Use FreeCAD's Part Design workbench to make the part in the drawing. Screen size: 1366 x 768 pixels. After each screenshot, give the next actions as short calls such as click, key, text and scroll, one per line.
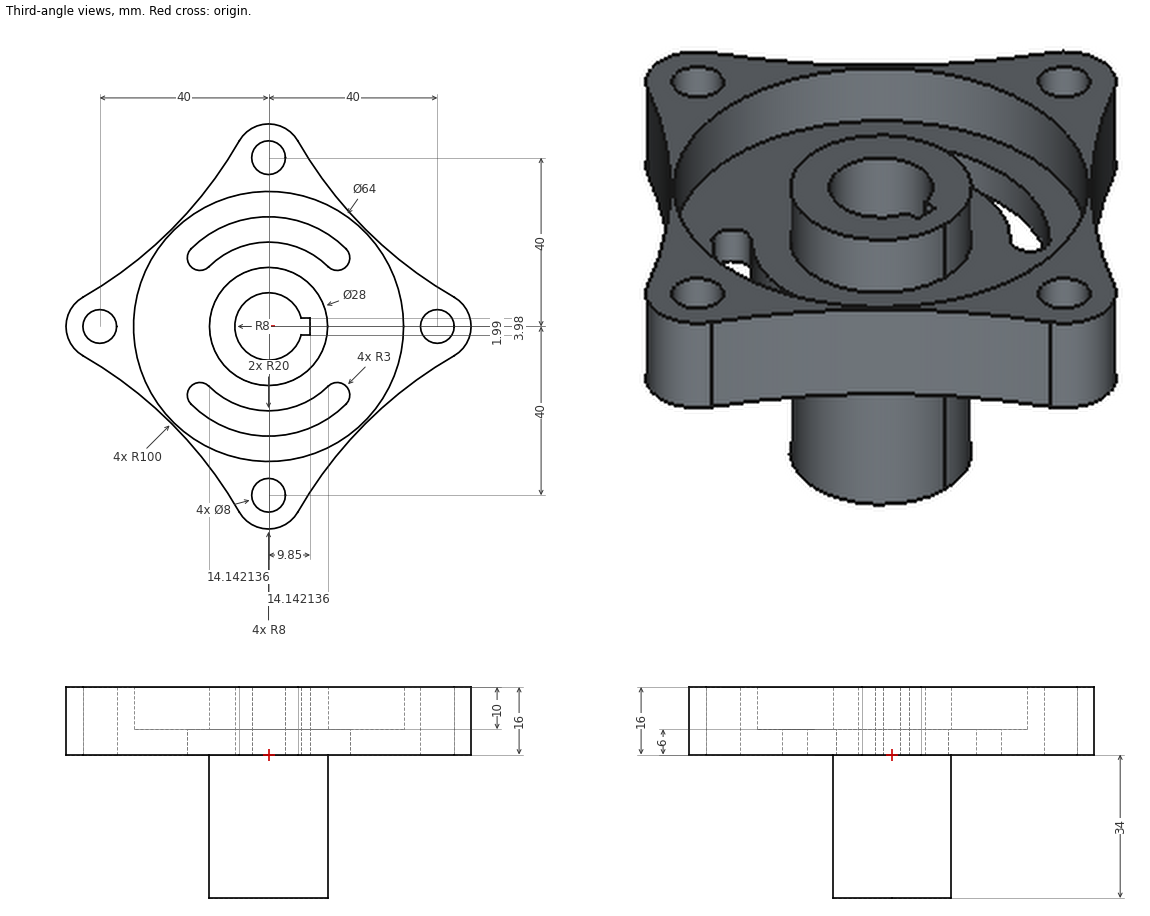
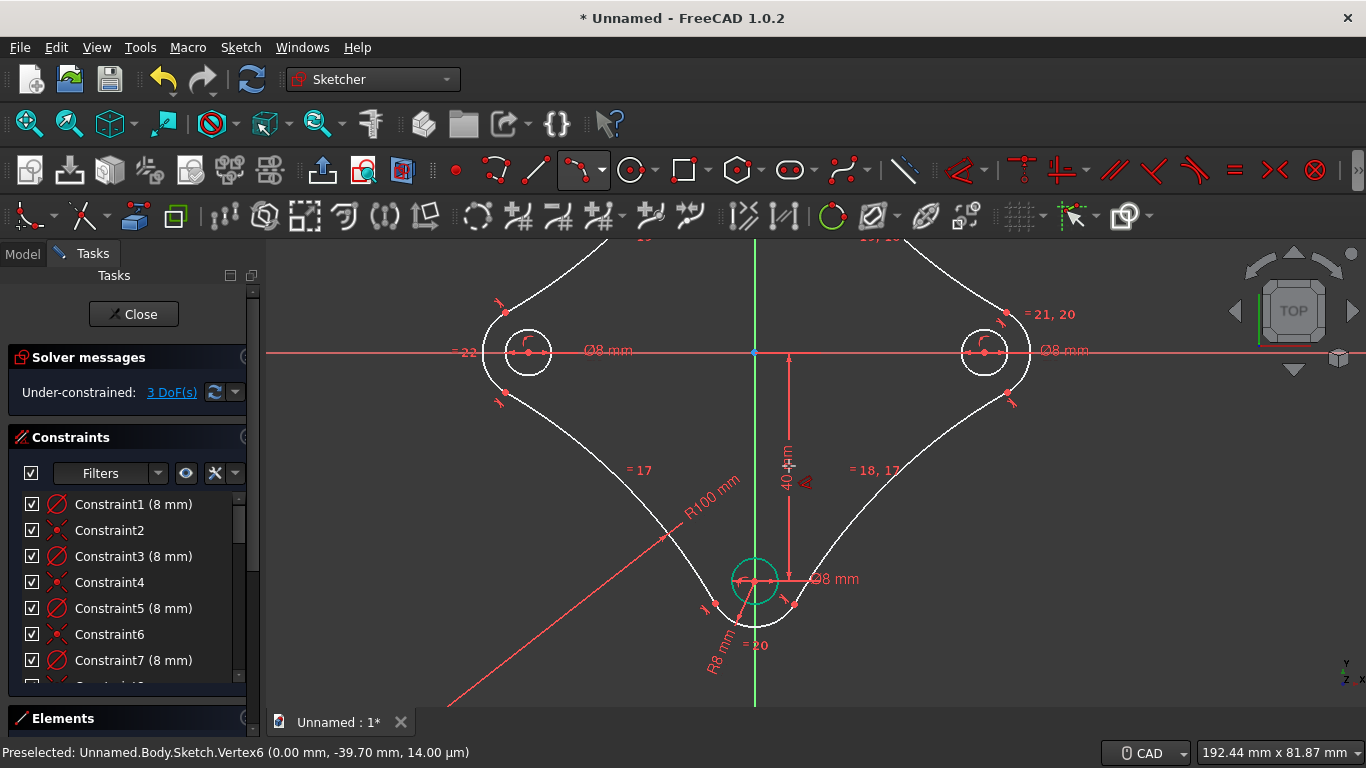
click(985, 353)
click(870, 387)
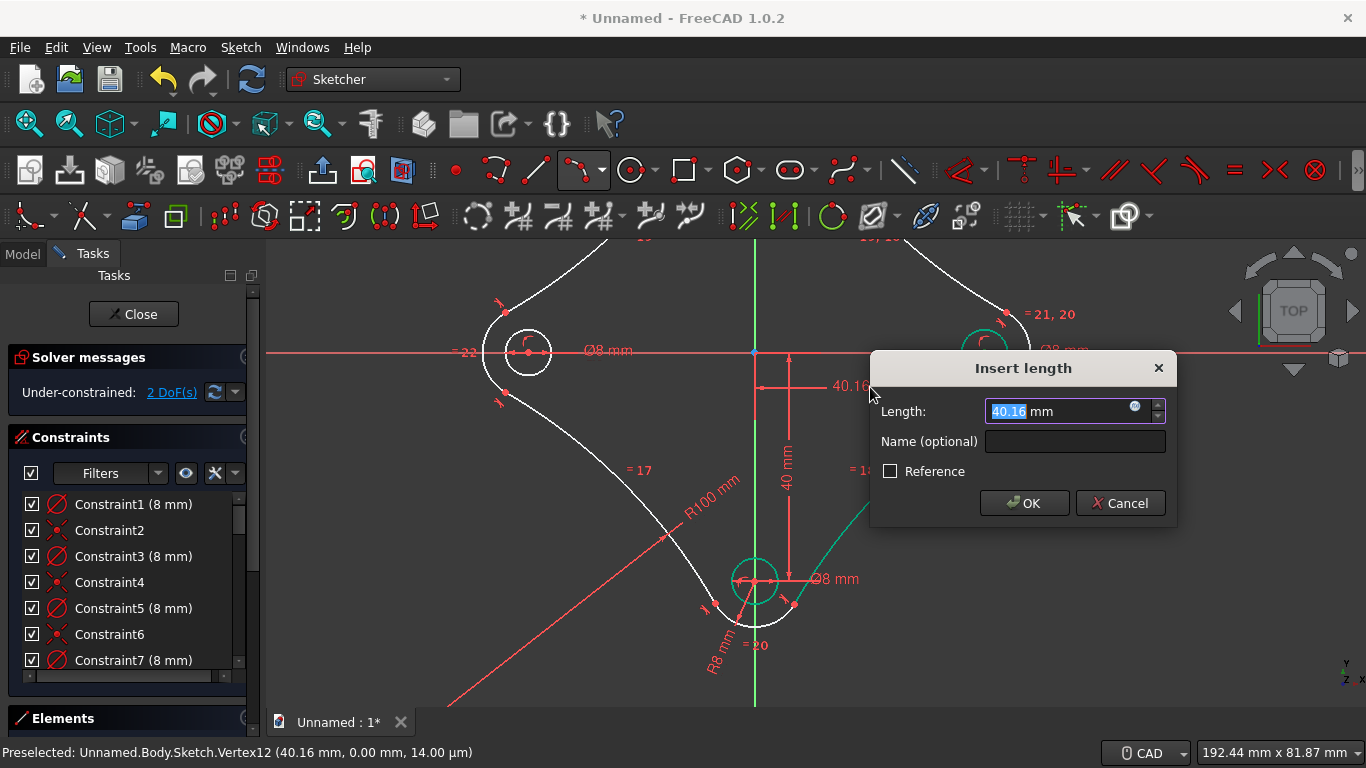
text(40)
key(Return)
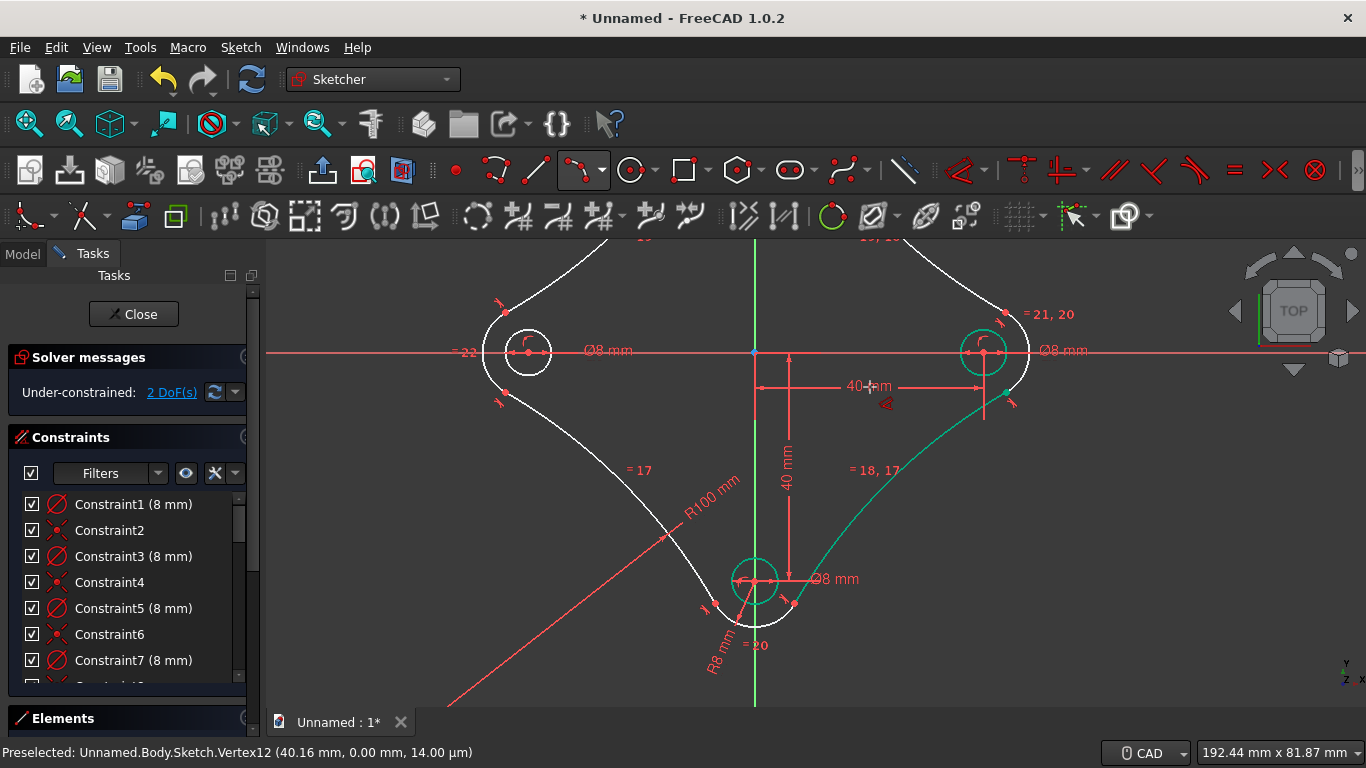
click(528, 353)
click(642, 387)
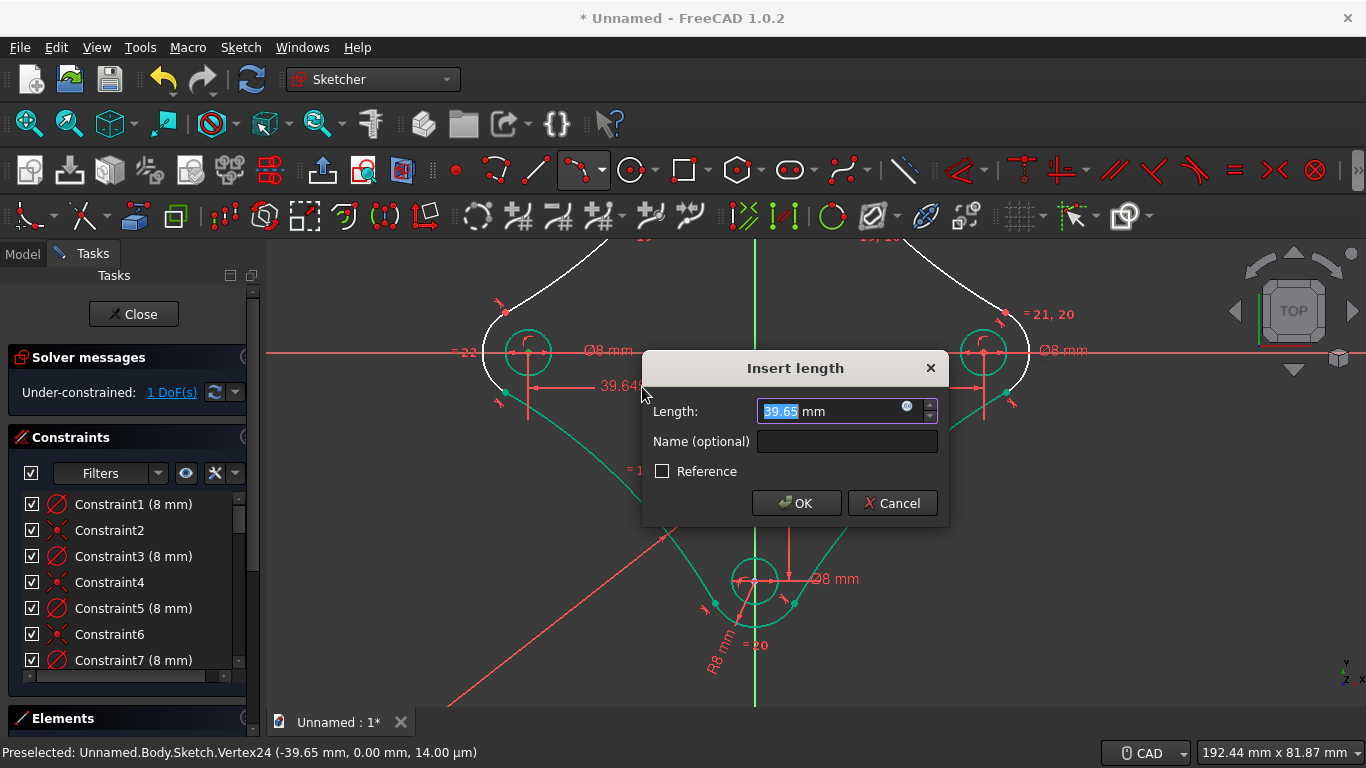
text(40)
key(Return)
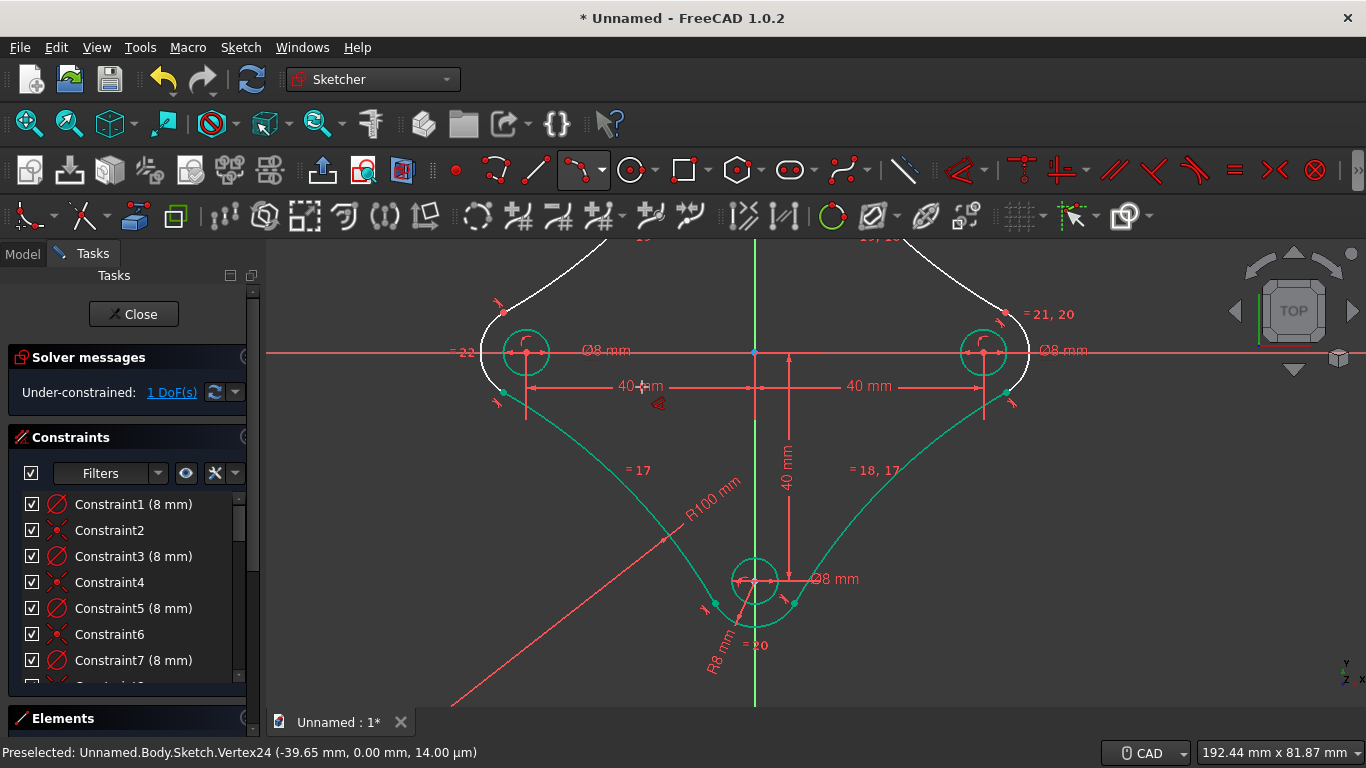
scroll(738, 619, down, 3)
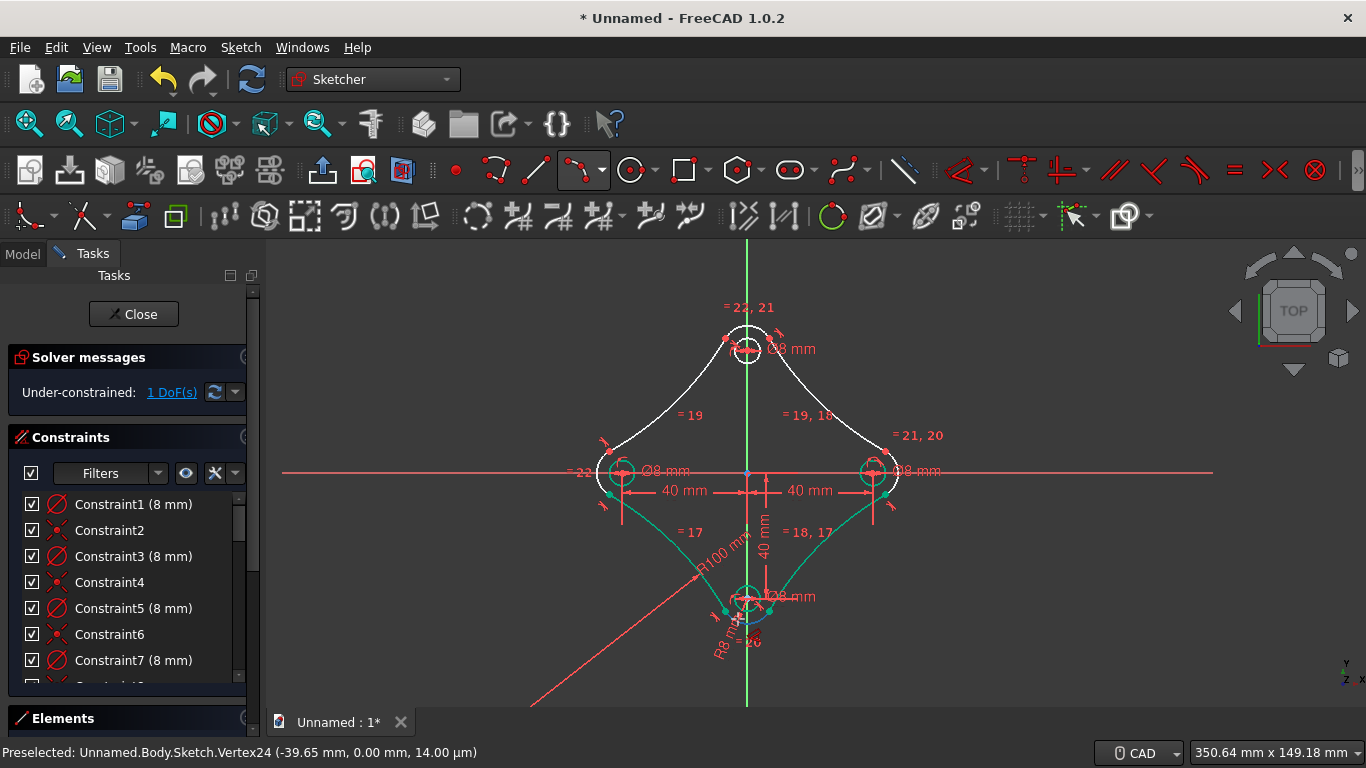
click(747, 351)
click(781, 412)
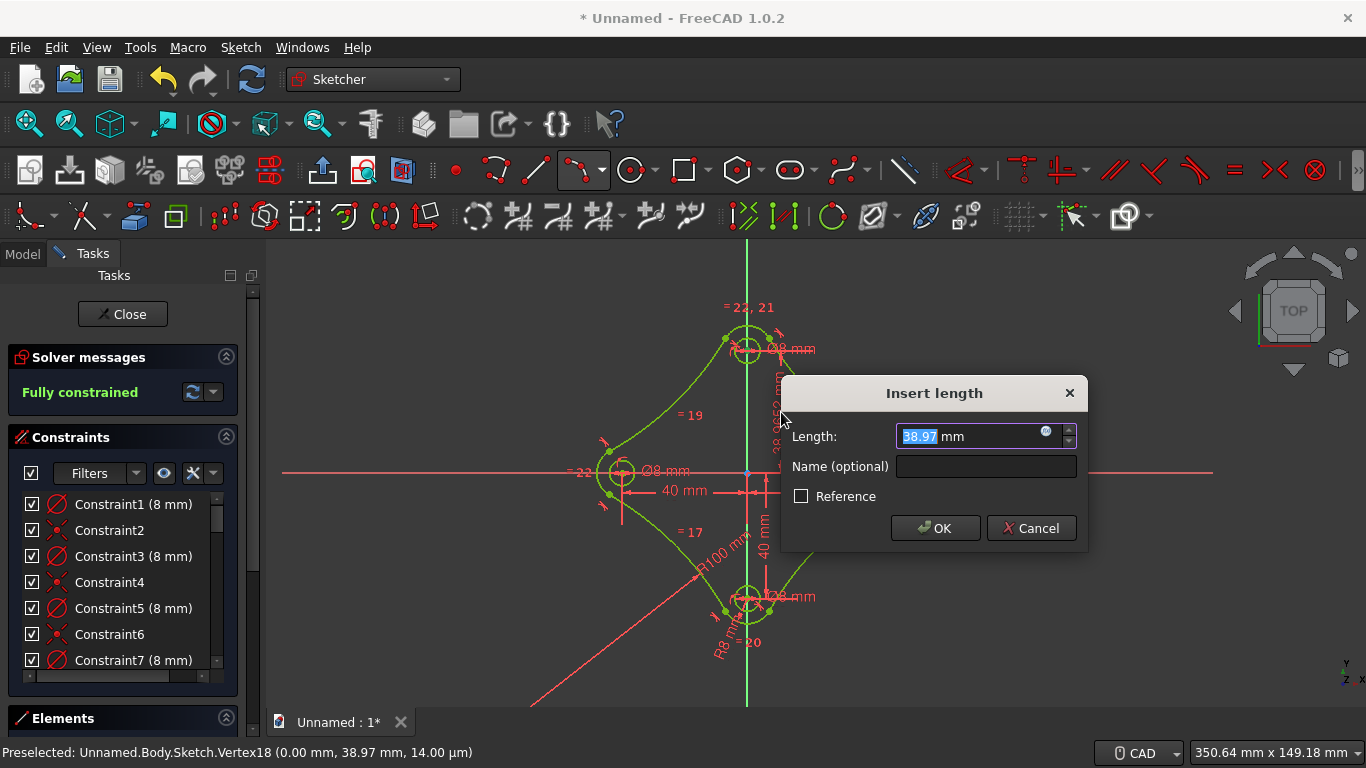
text(40)
key(Return)
key(Escape)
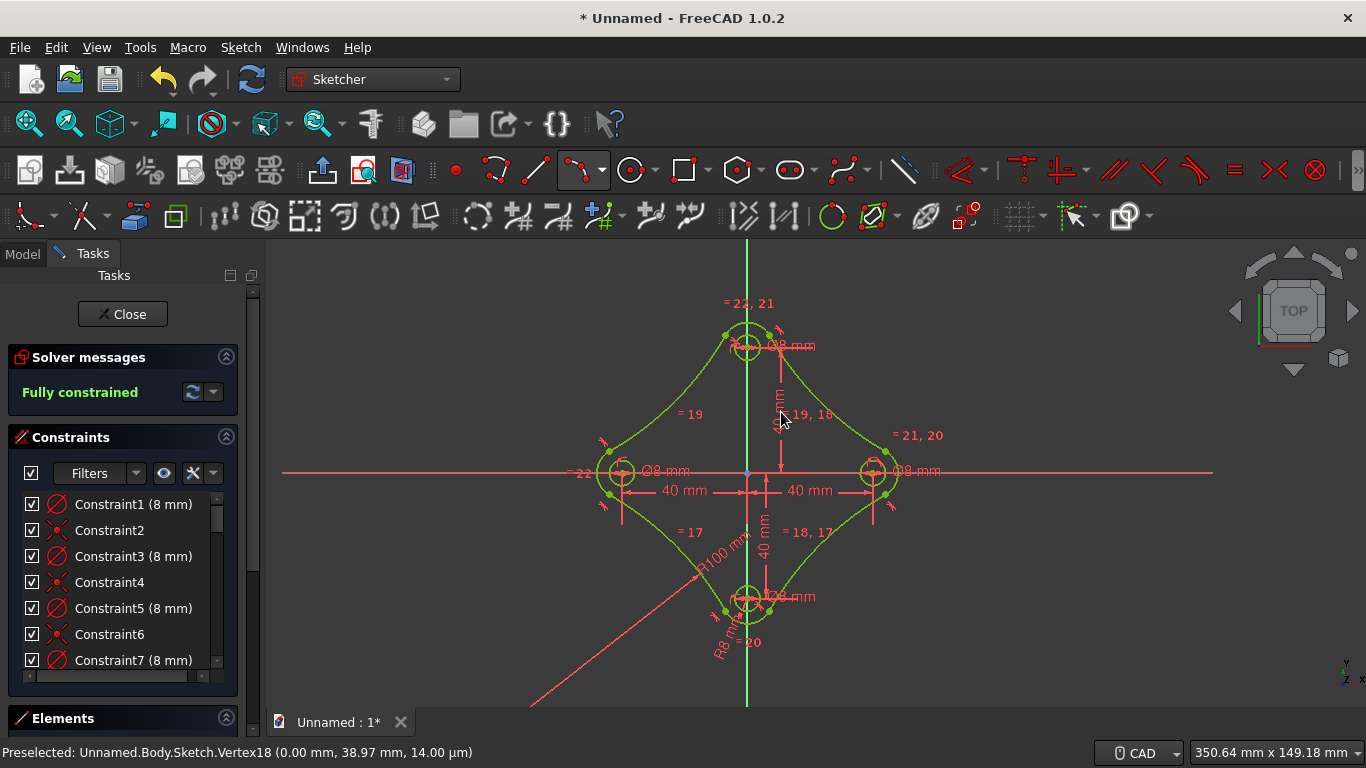
click(123, 314)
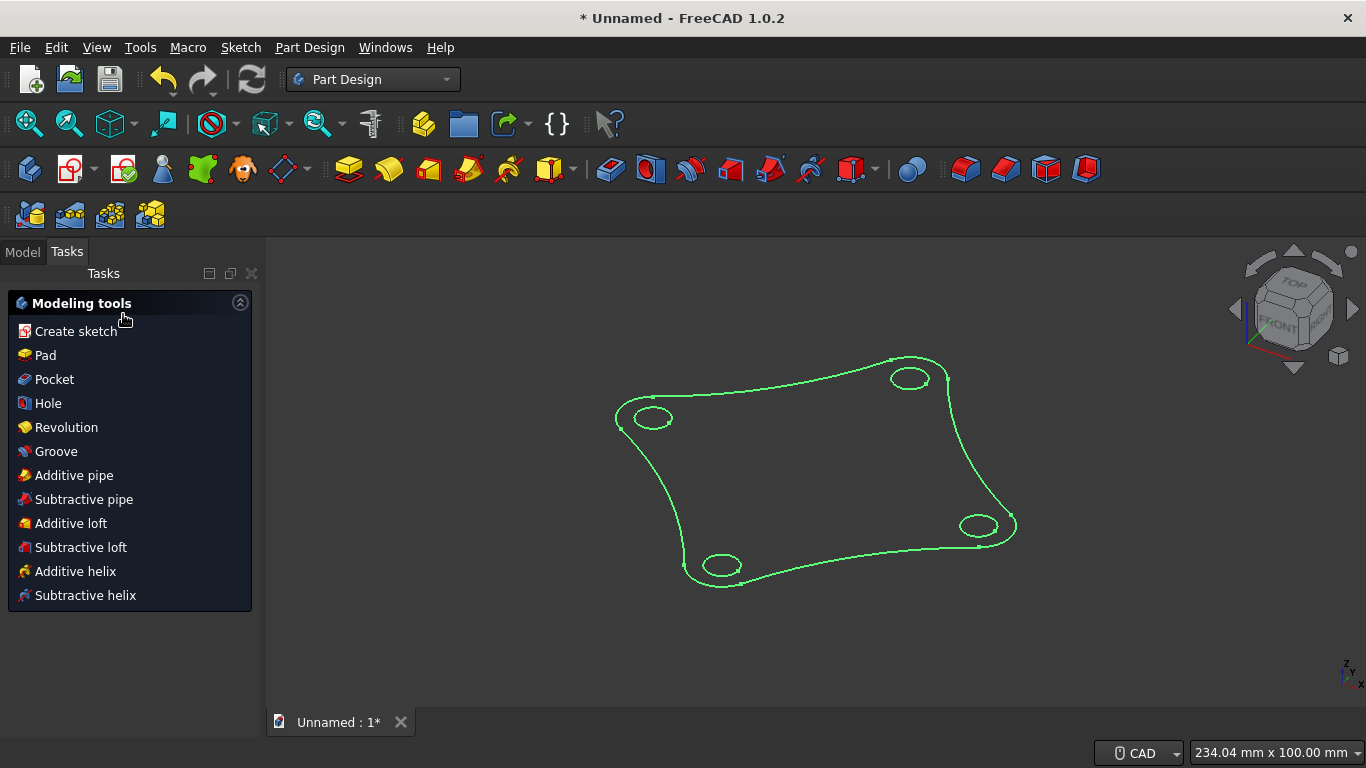
click(350, 170)